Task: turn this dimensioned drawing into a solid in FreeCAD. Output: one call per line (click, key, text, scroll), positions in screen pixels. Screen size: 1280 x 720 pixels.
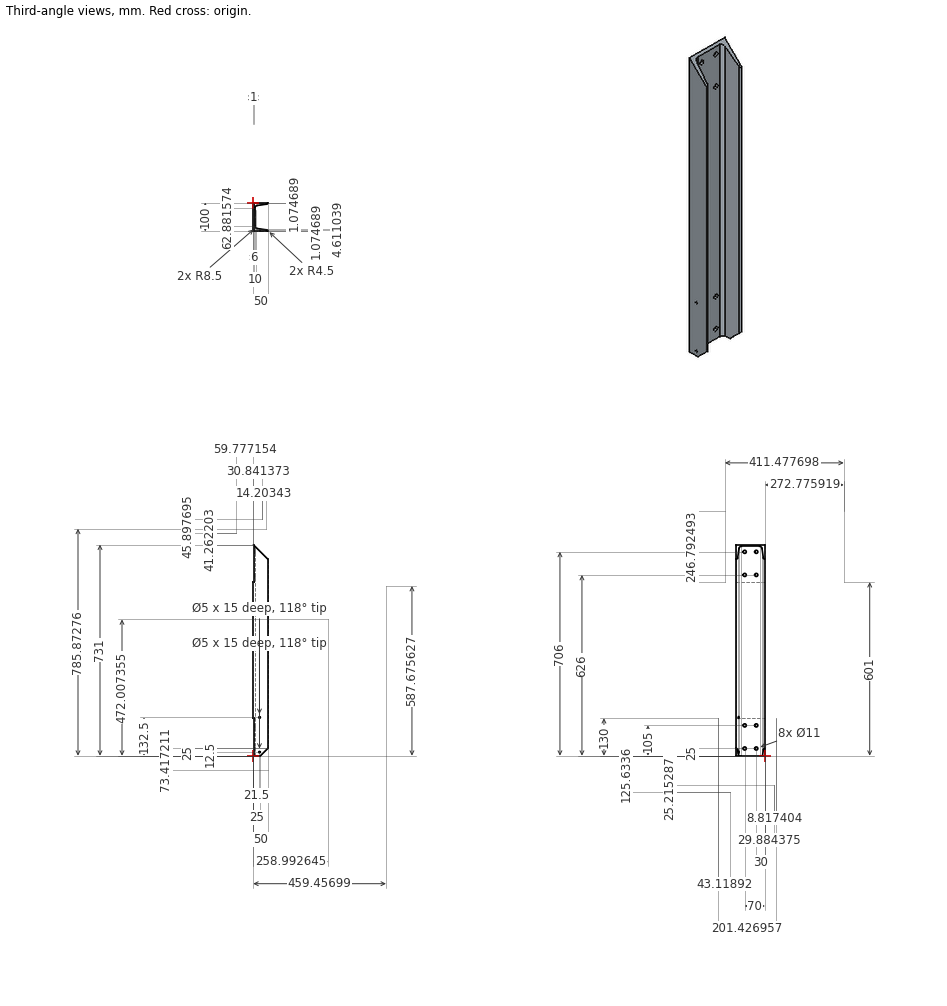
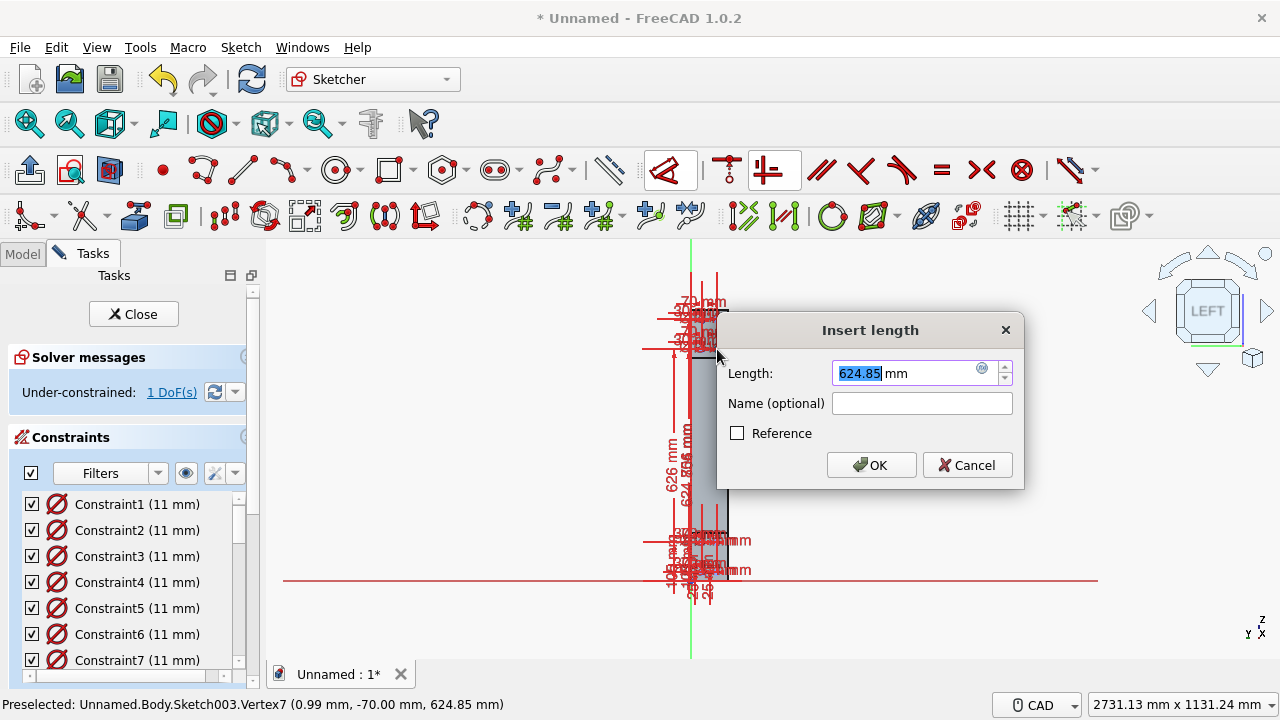
text(626)
key(Return)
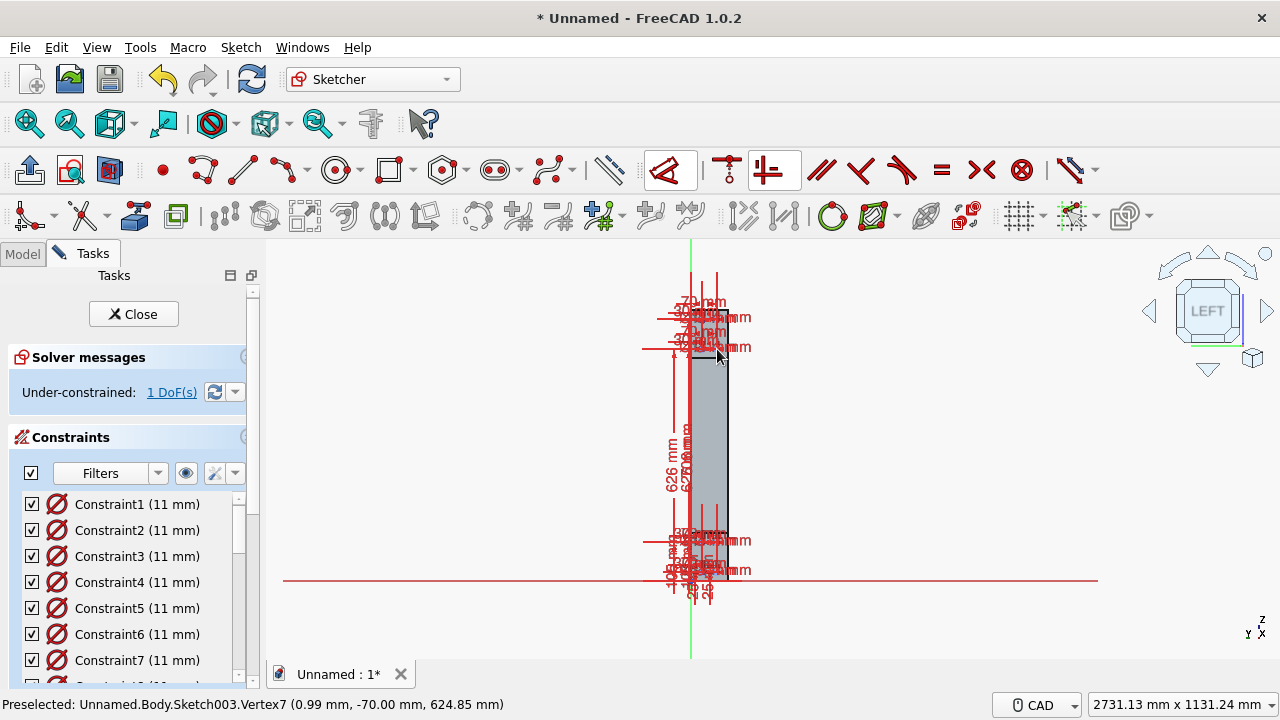
click(702, 320)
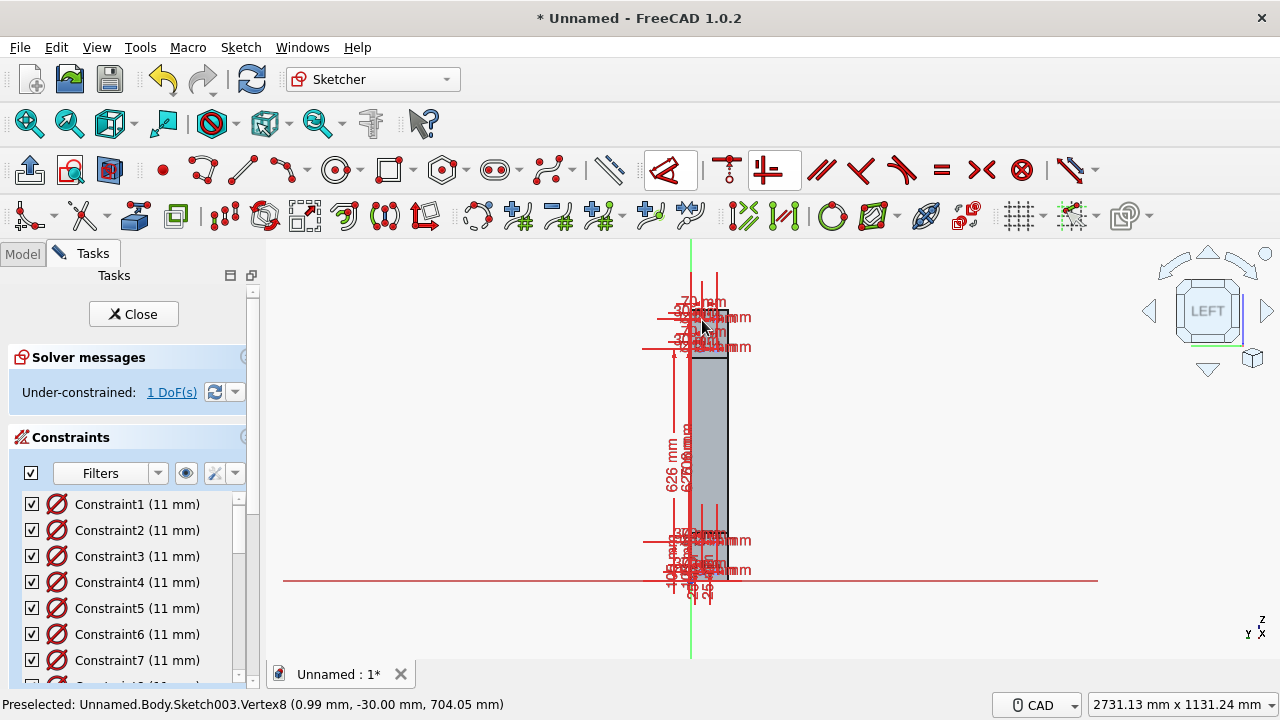
key(i)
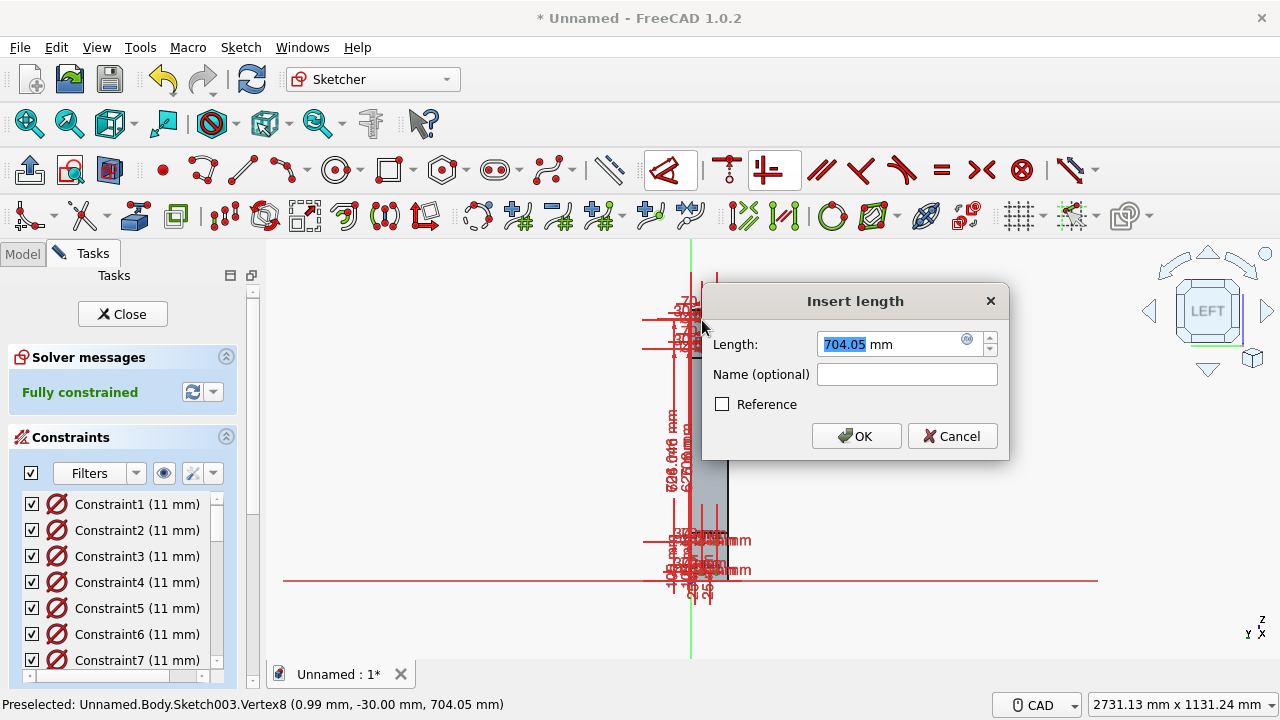
text(706)
key(Return)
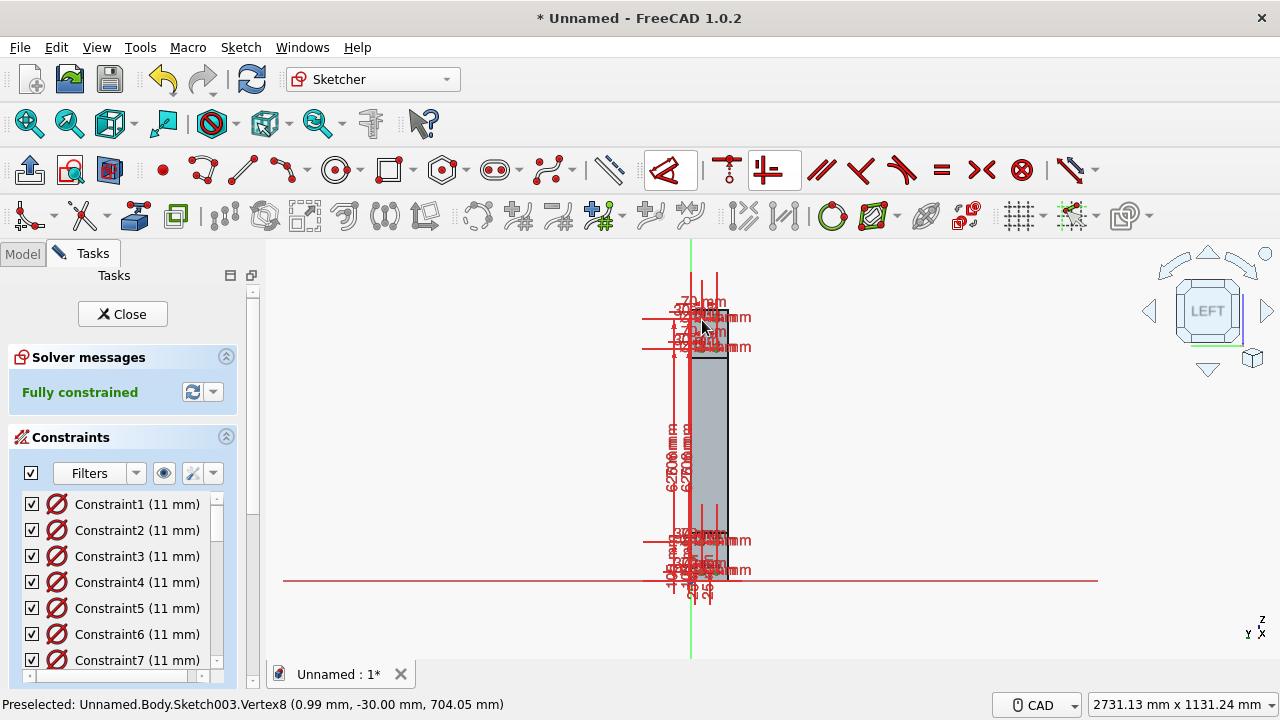
click(123, 314)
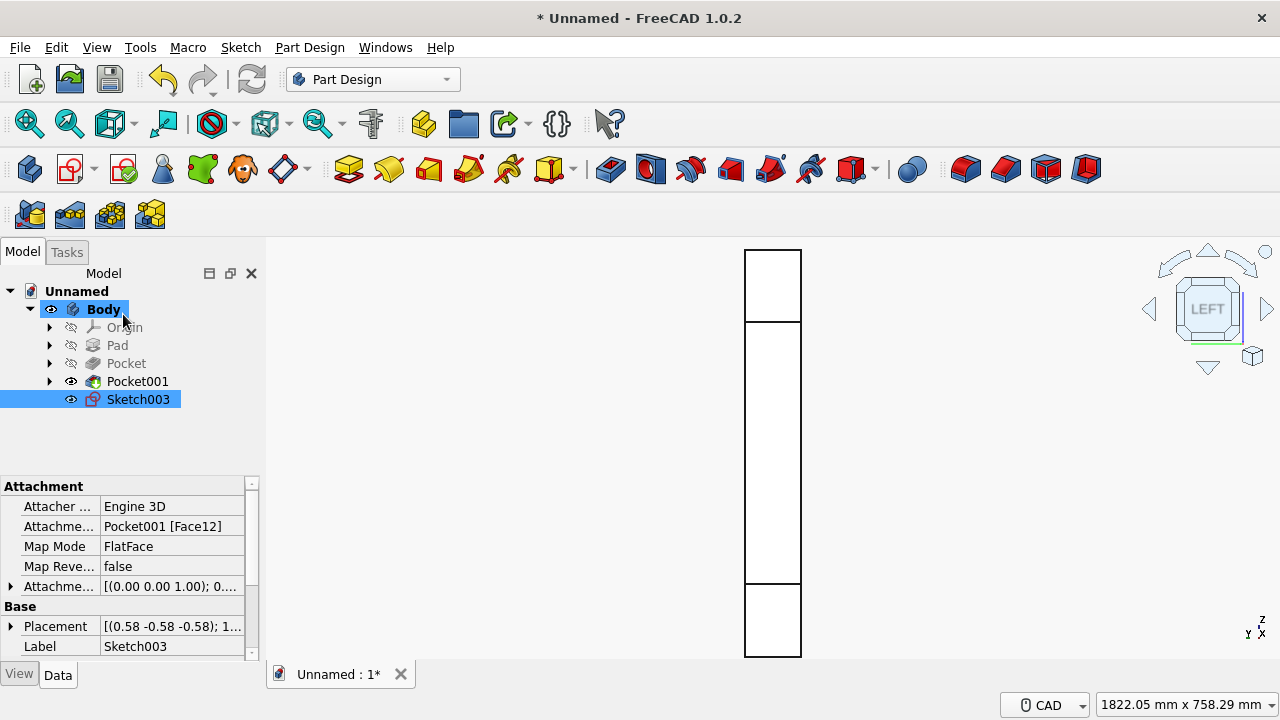
click(612, 170)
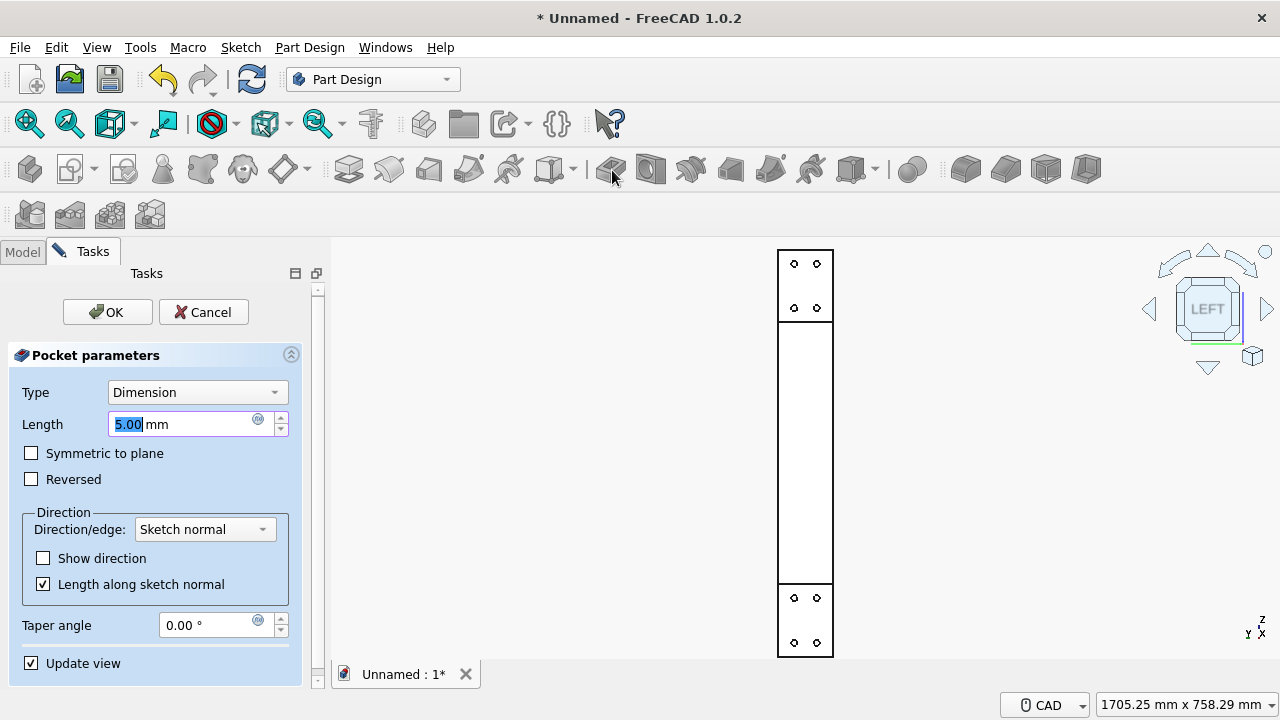
text(10)
key(Tab)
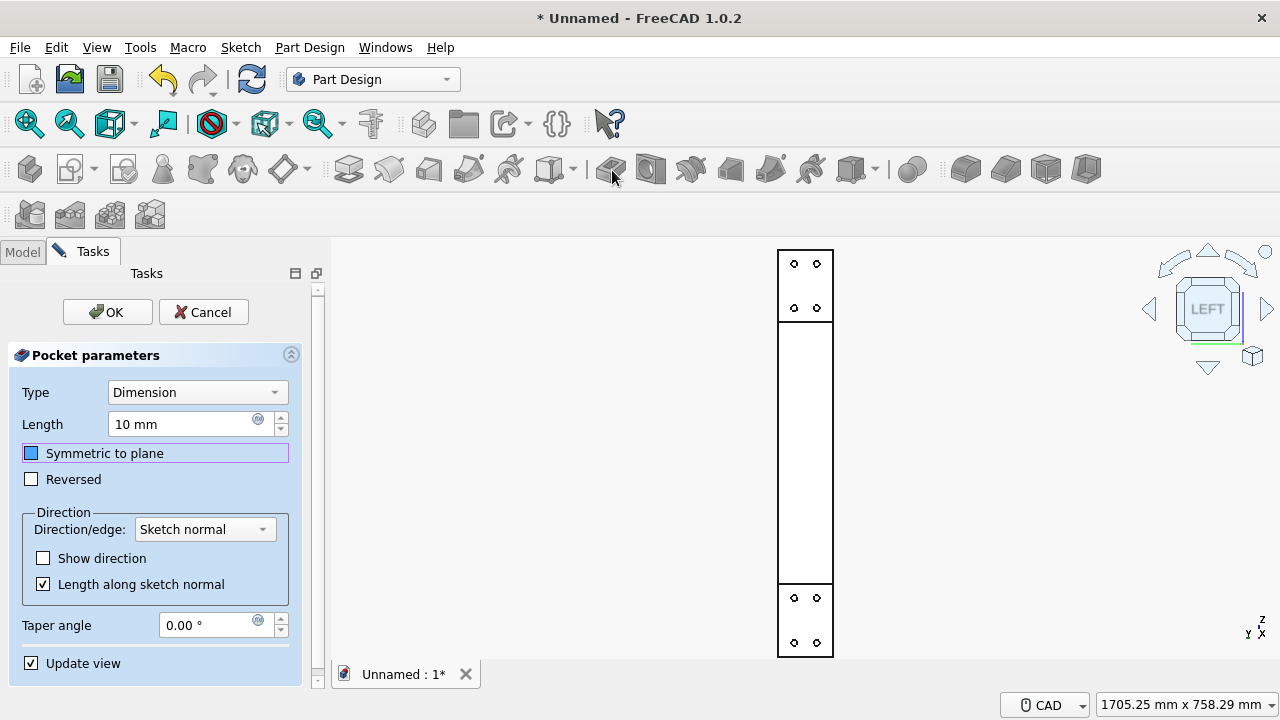
click(108, 312)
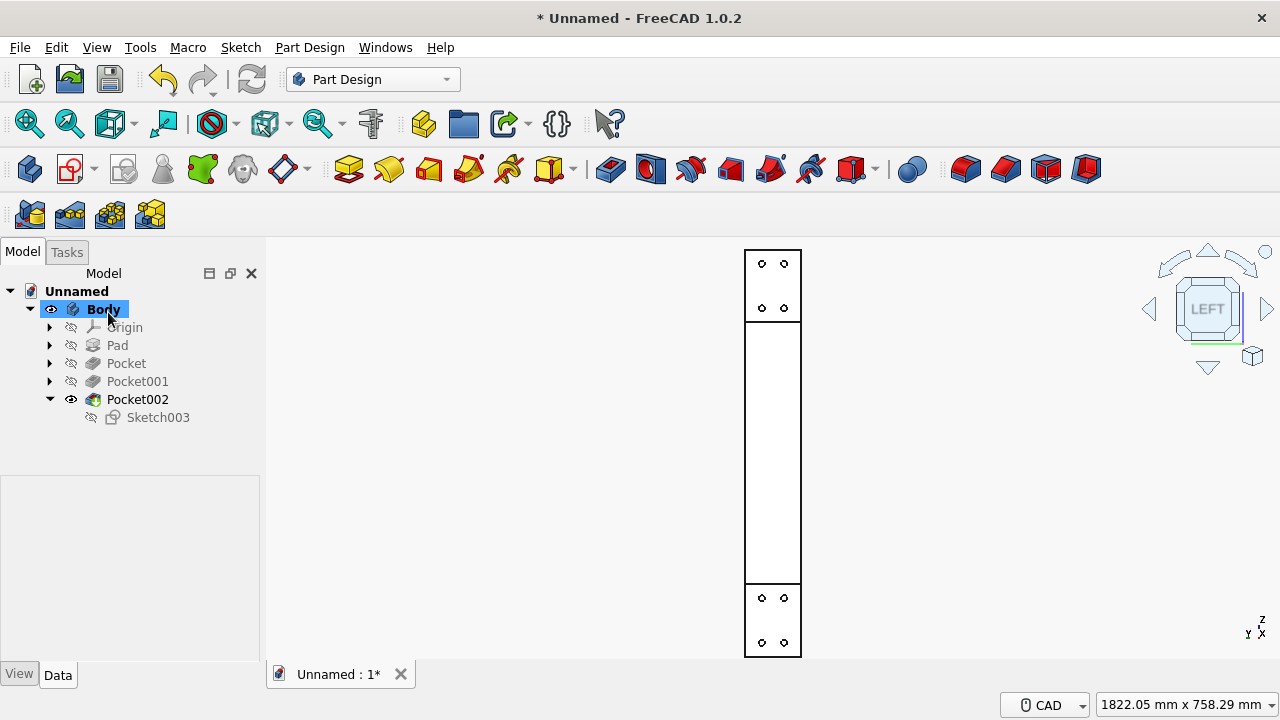
key(0)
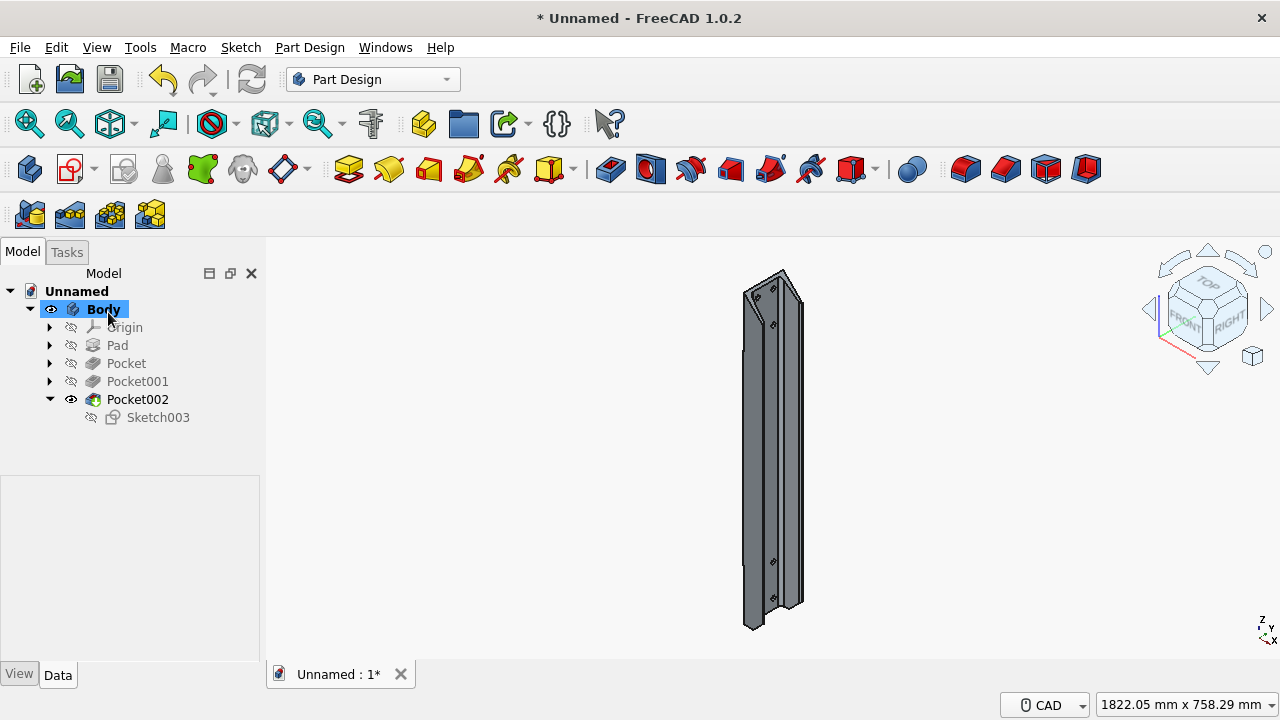
click(753, 368)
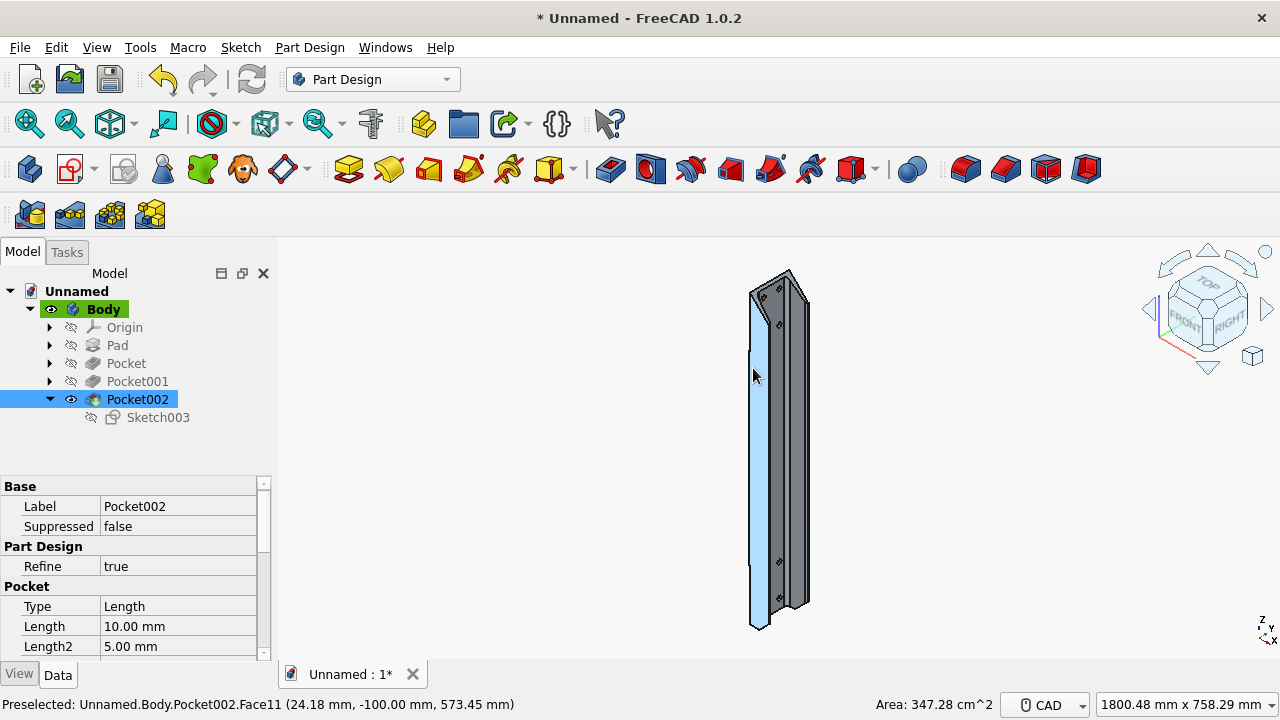
click(70, 170)